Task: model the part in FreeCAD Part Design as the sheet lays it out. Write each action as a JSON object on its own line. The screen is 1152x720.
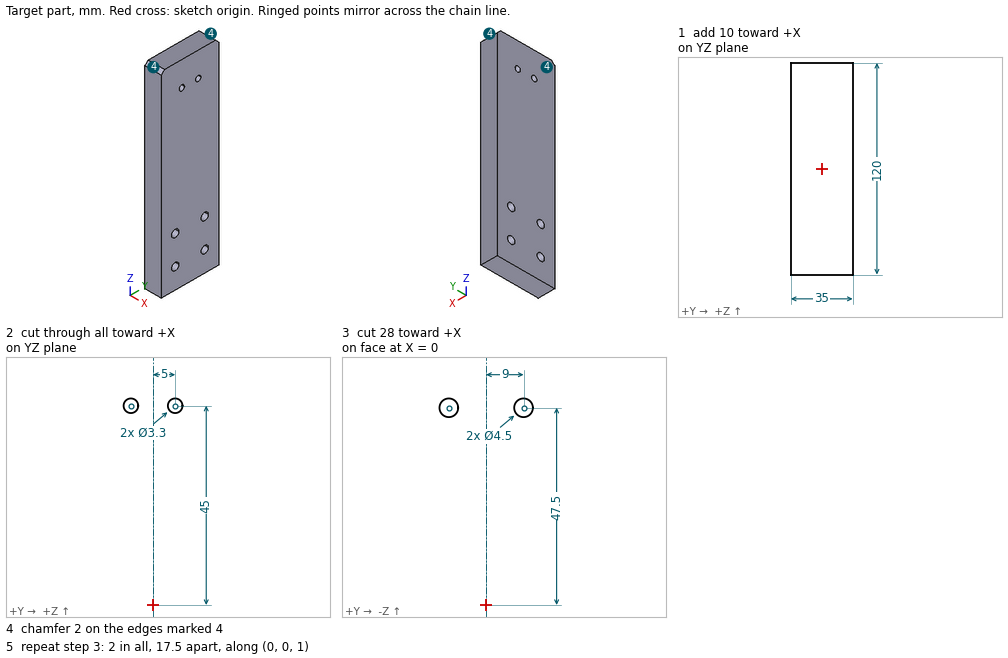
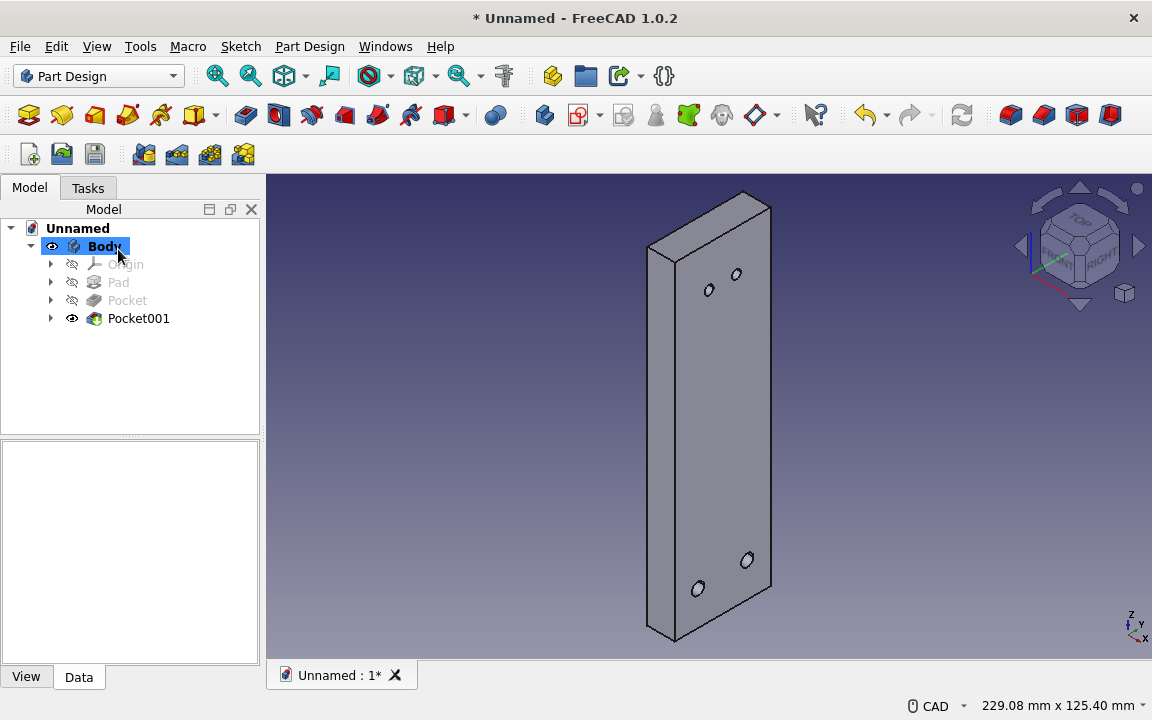
{"action": "left_click", "coordinate": [661, 254]}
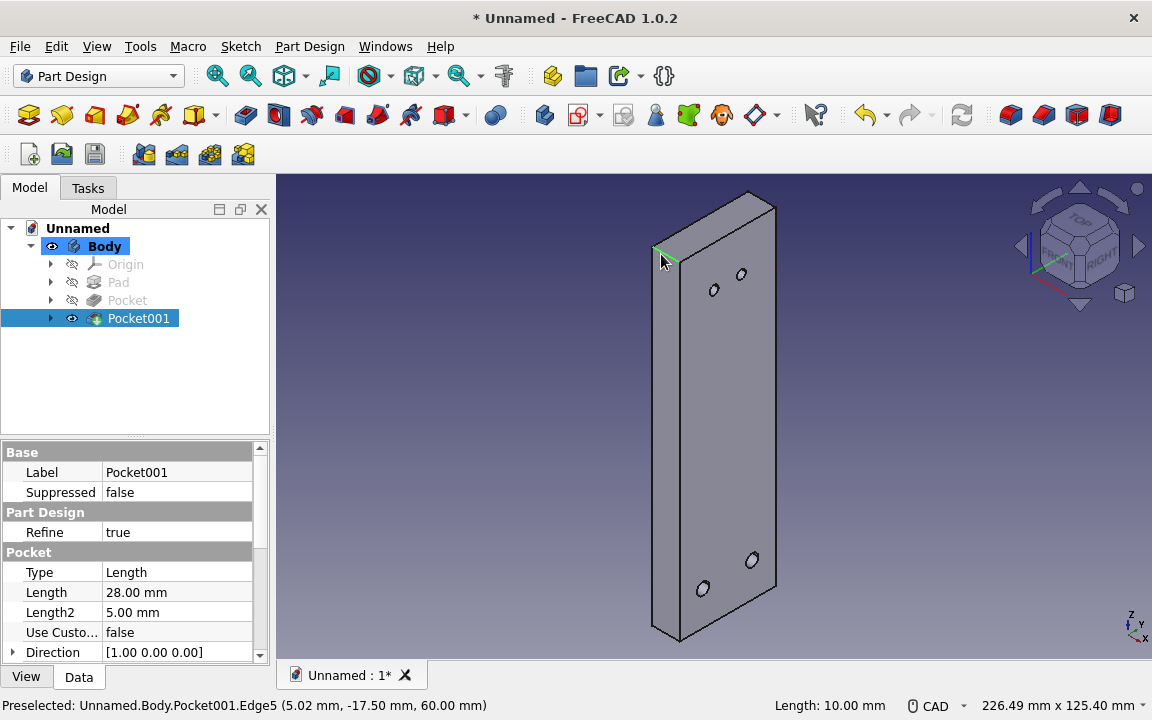
{"action": "key", "text": "2"}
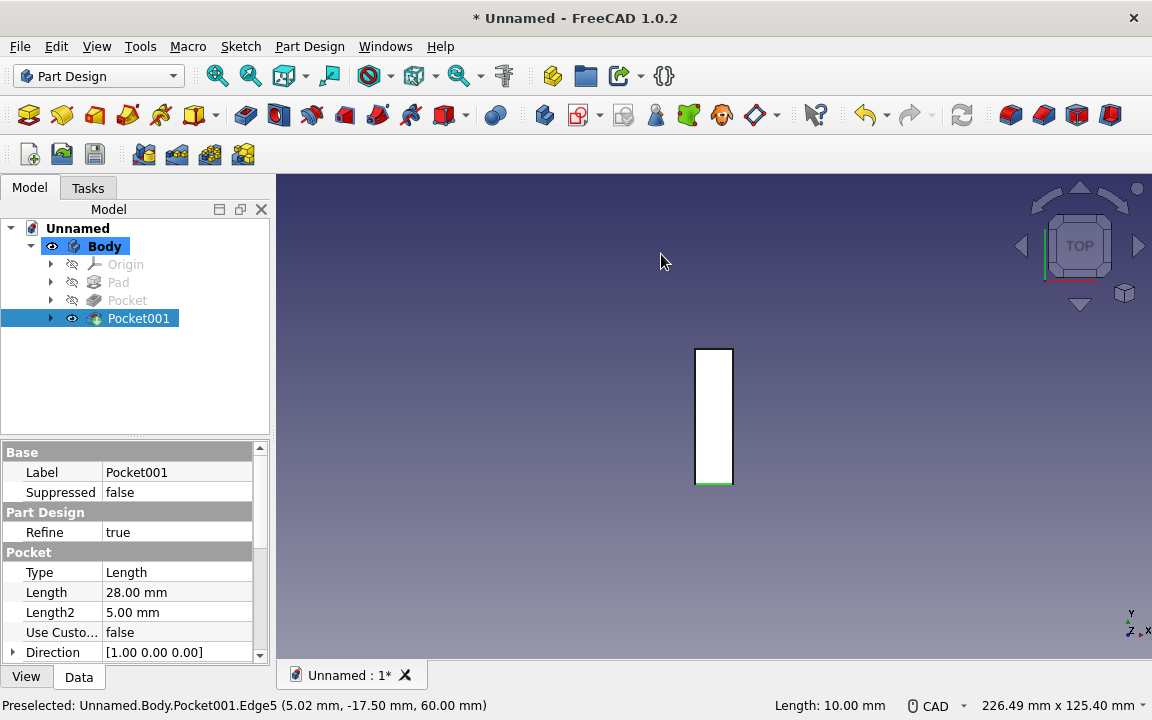
{"action": "left_click", "coordinate": [218, 76]}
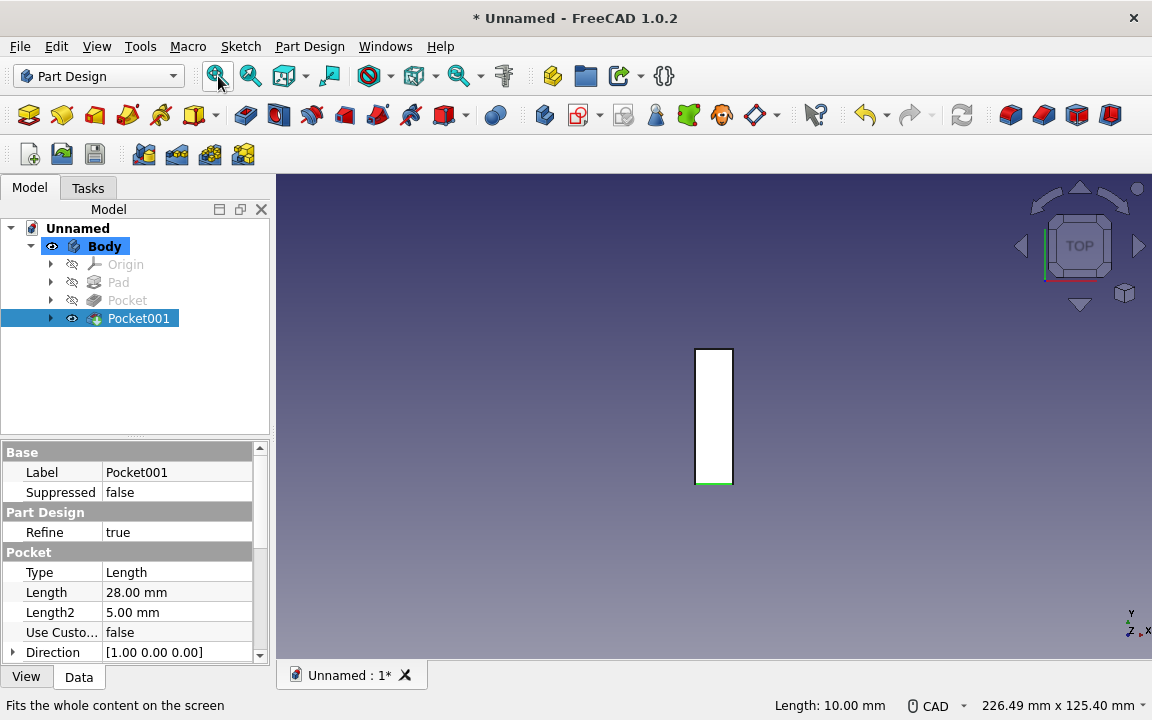
{"action": "left_click", "coordinate": [714, 348], "text": "ctrl"}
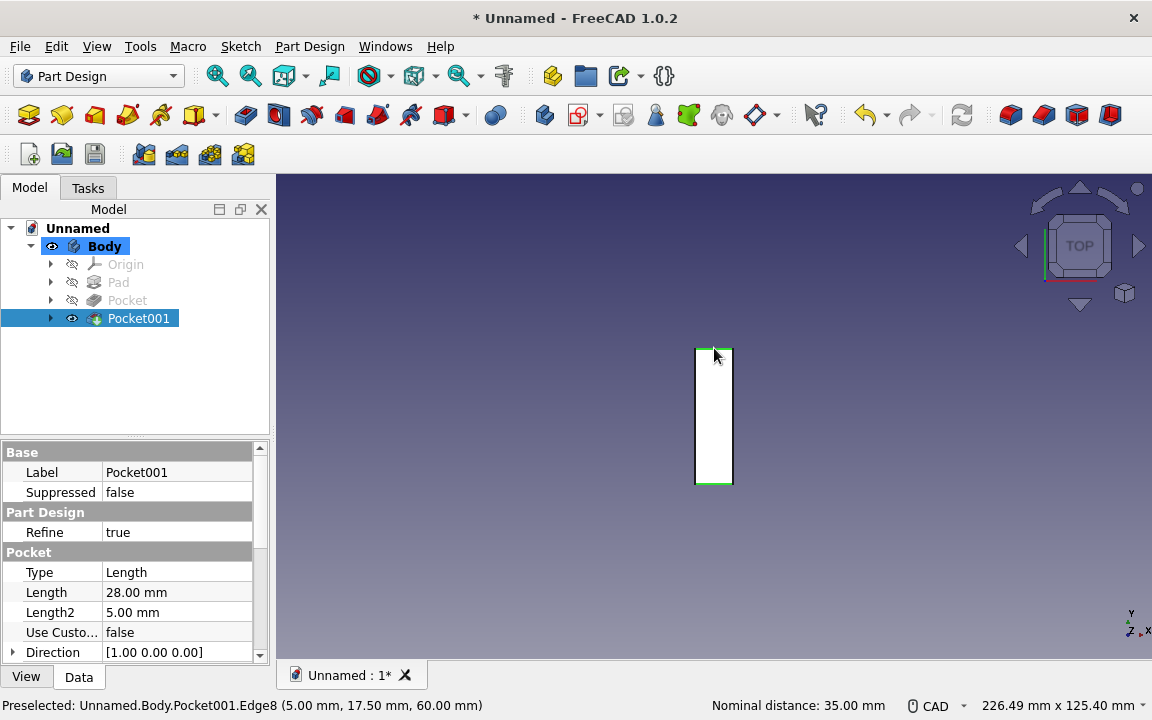
{"action": "left_click", "coordinate": [1044, 116]}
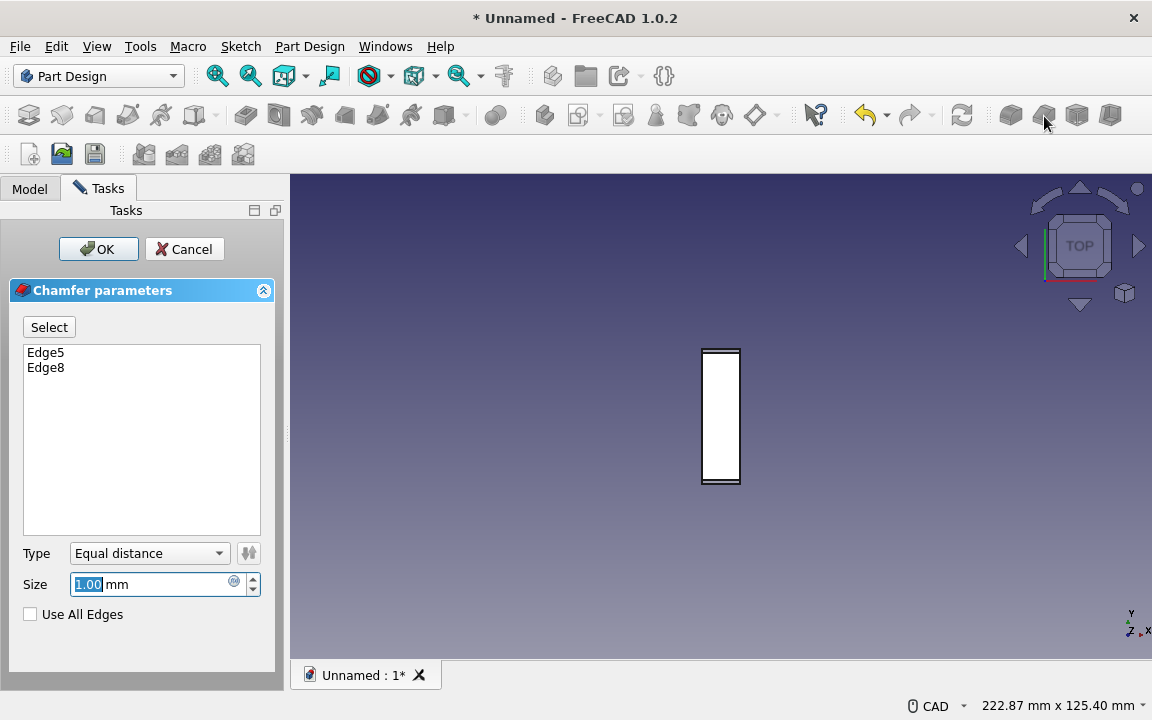
{"action": "type", "text": "2"}
{"action": "key", "text": "Tab"}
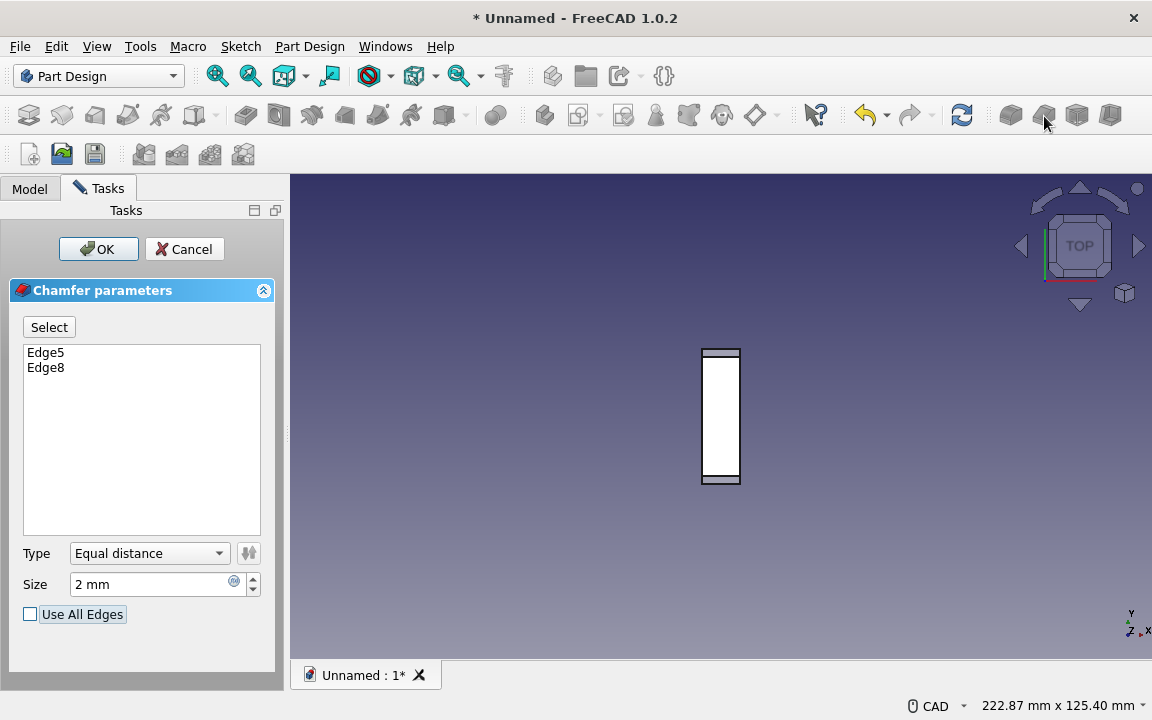
{"action": "left_click", "coordinate": [99, 249]}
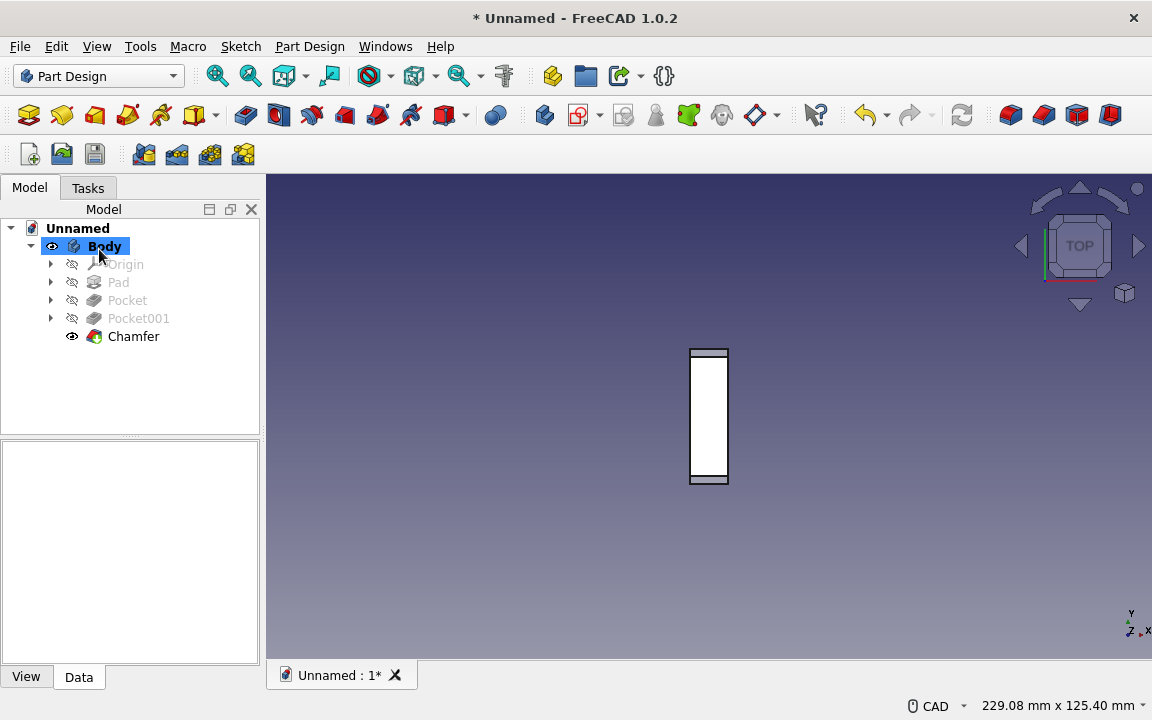
{"action": "left_click", "coordinate": [218, 76]}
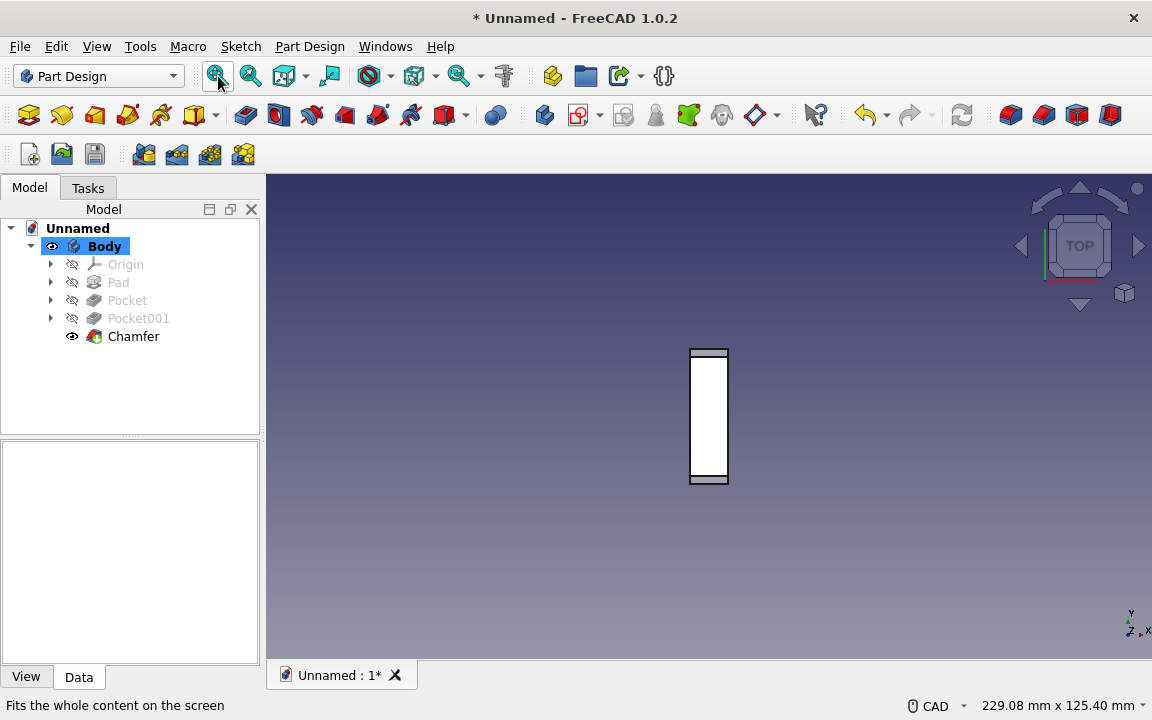
{"action": "left_click", "coordinate": [117, 318]}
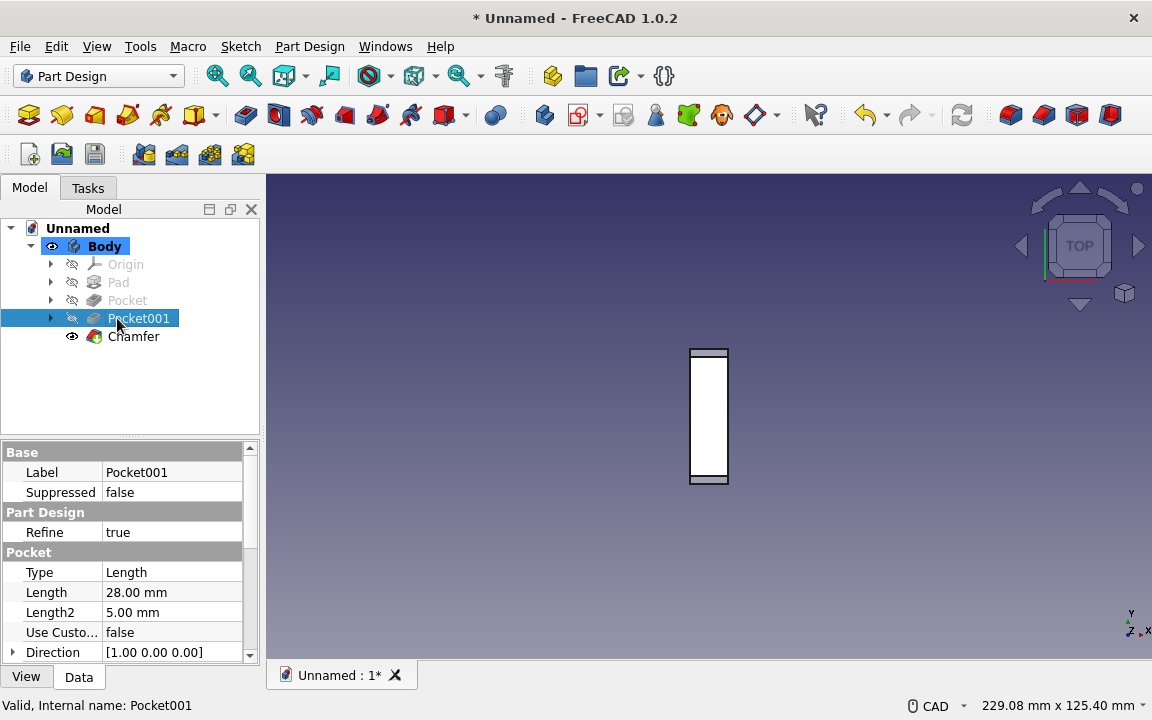
{"action": "left_click", "coordinate": [177, 154]}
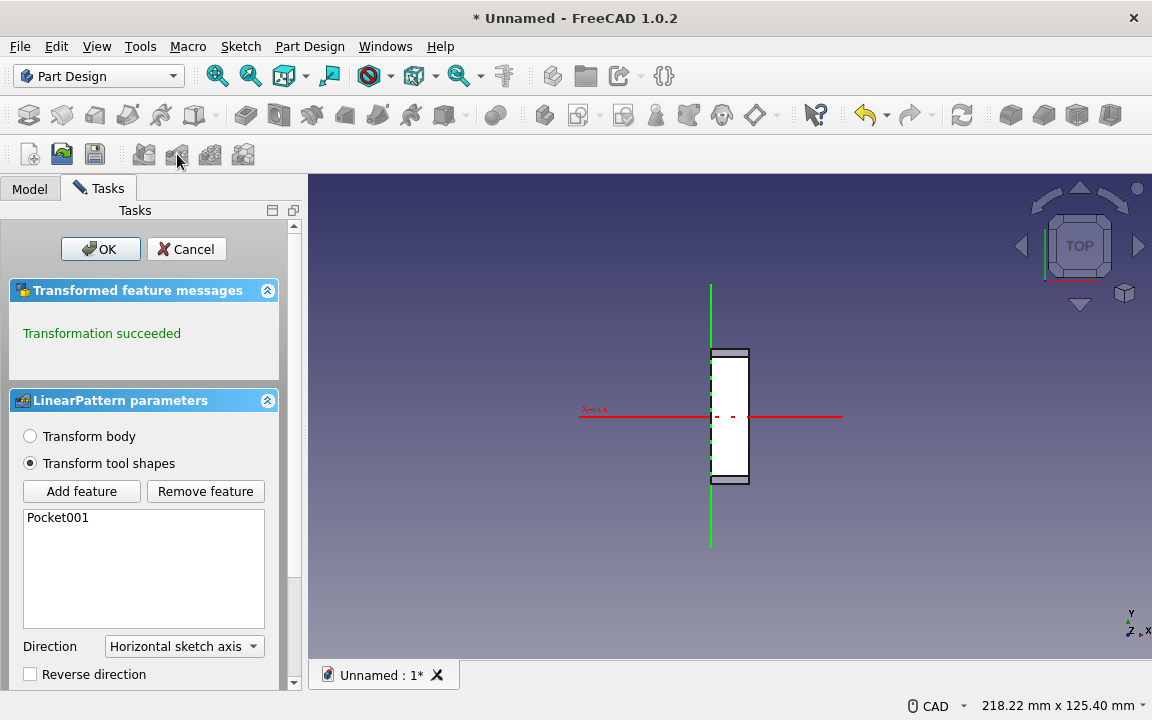
{"action": "left_click", "coordinate": [185, 646]}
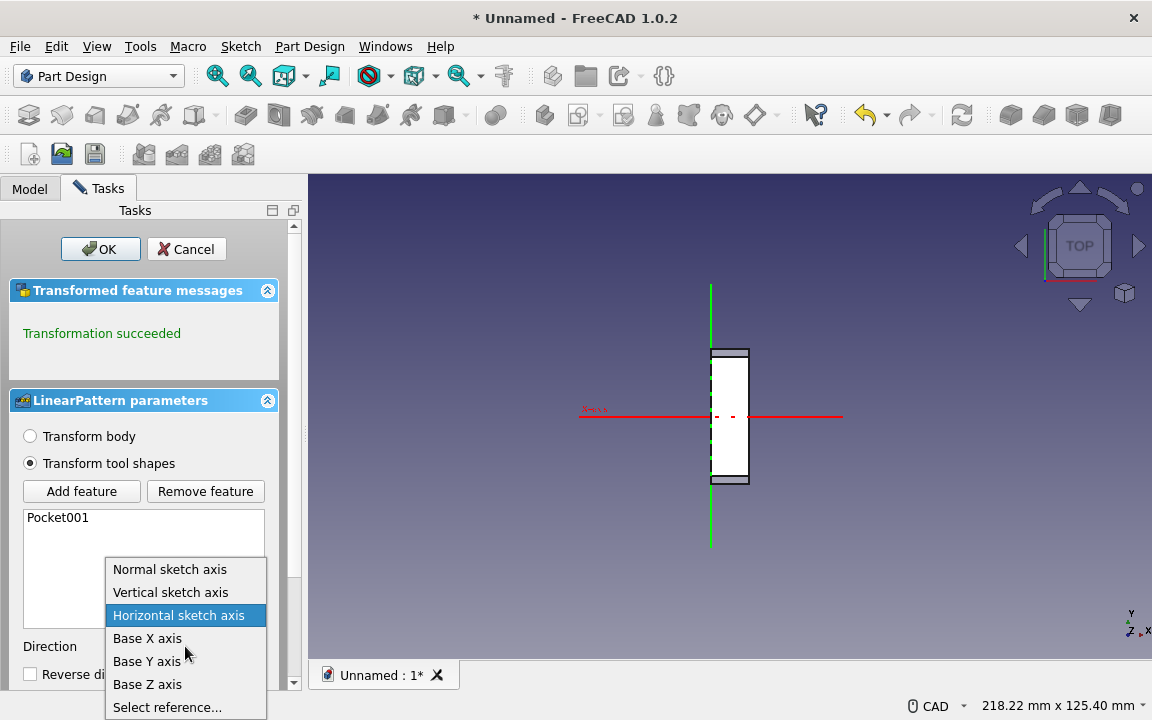
{"action": "left_click", "coordinate": [184, 684]}